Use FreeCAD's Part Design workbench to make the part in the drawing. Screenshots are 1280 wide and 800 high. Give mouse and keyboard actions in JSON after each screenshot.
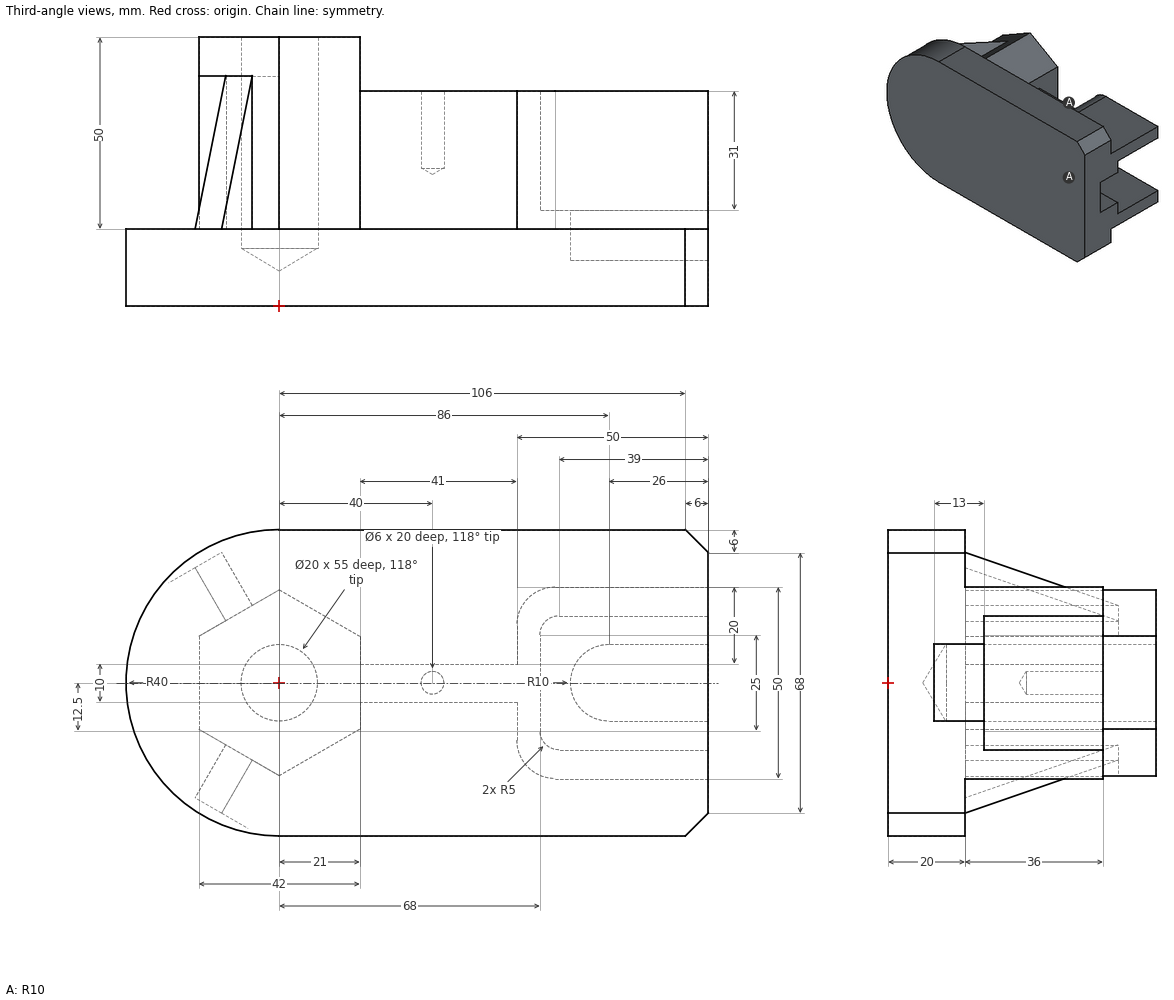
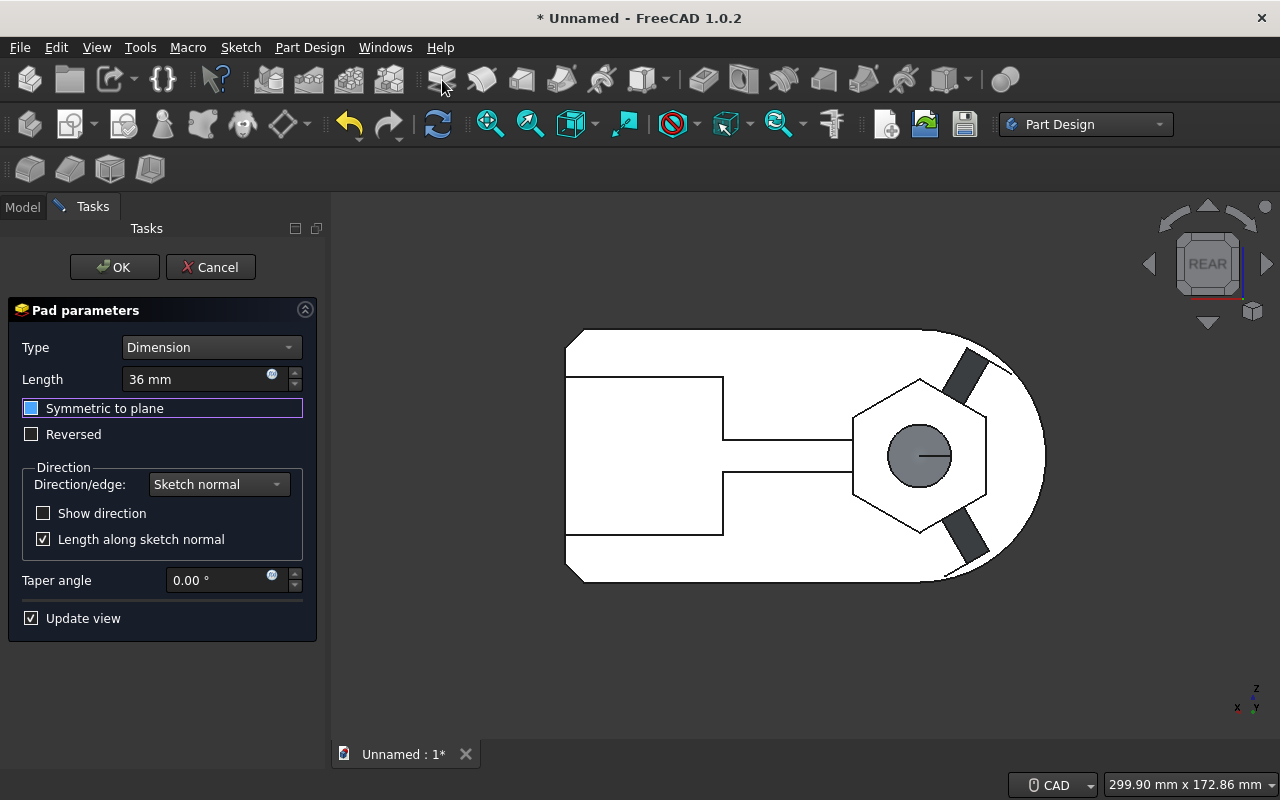
{"action": "left_click", "coordinate": [115, 267]}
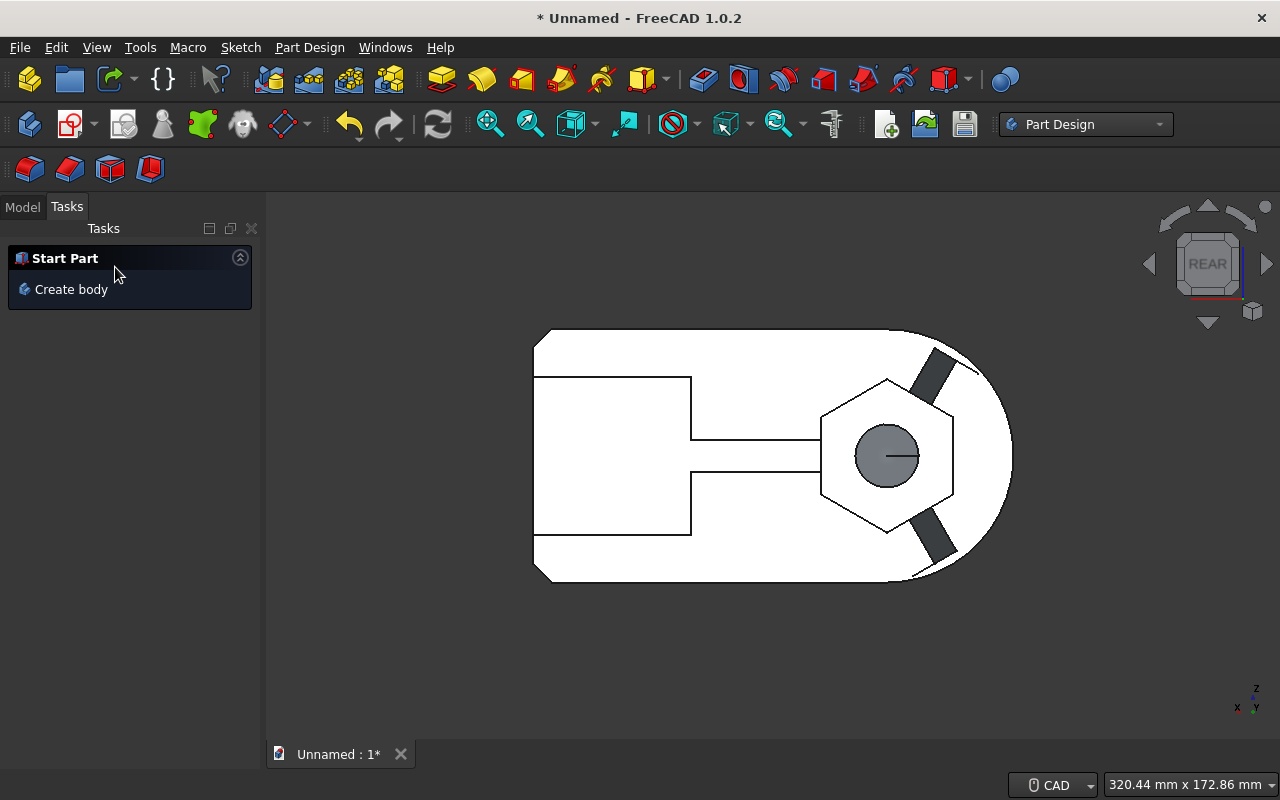
{"action": "key", "text": "0"}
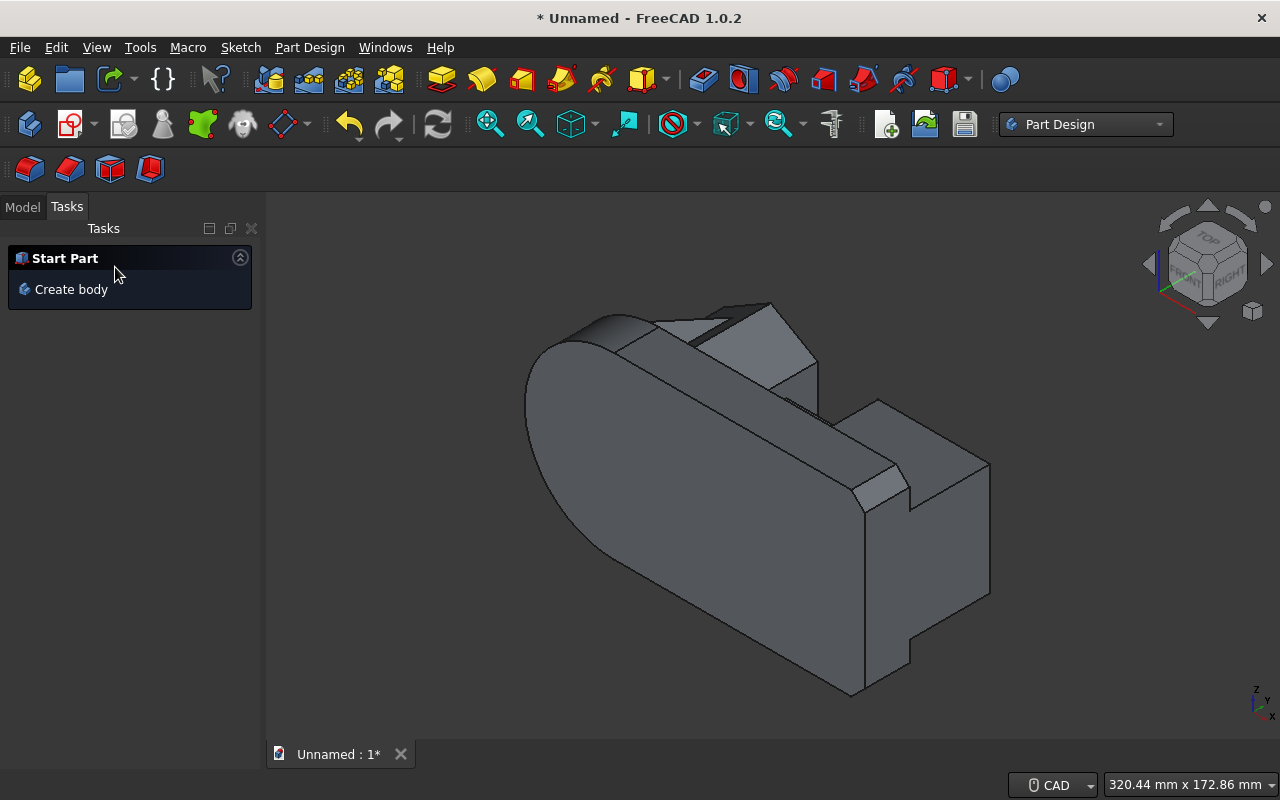
{"action": "key", "text": "2"}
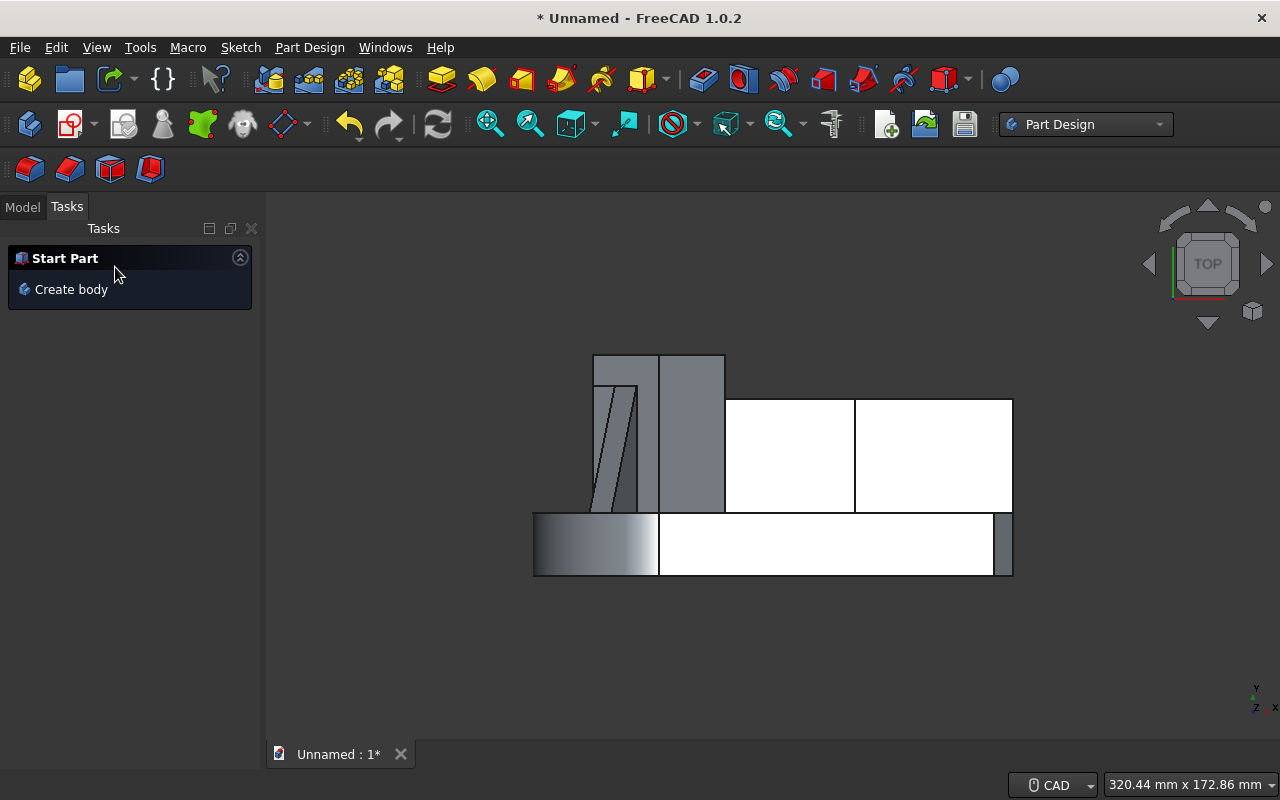
{"action": "left_click", "coordinate": [855, 455]}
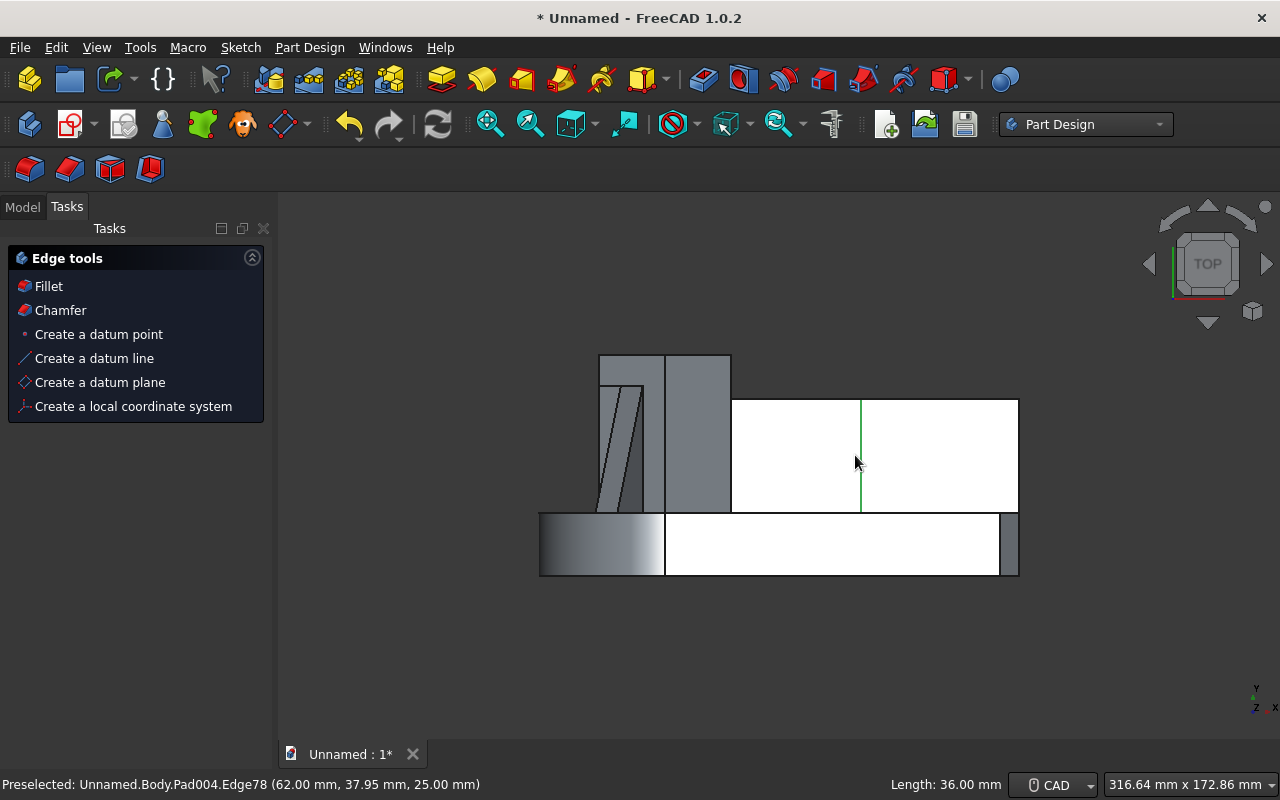
{"action": "key", "text": "1"}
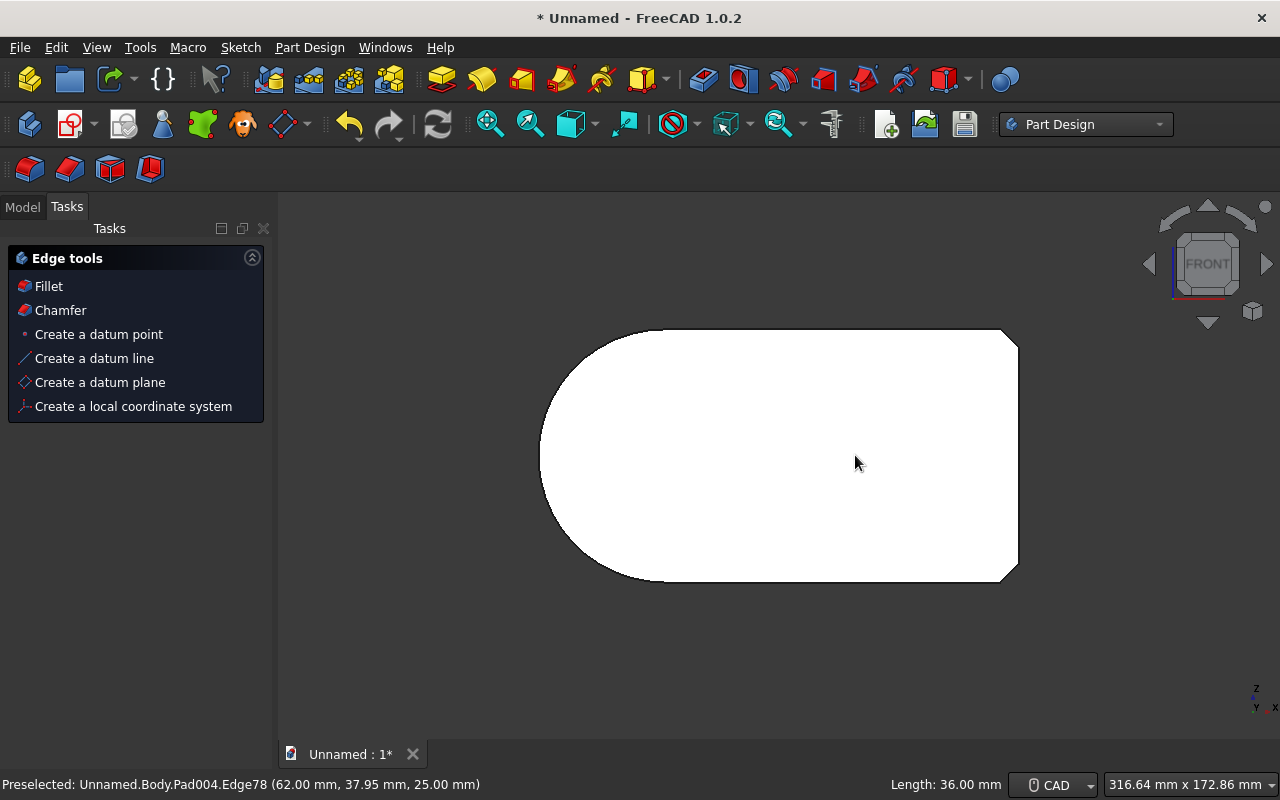
{"action": "key", "text": "3"}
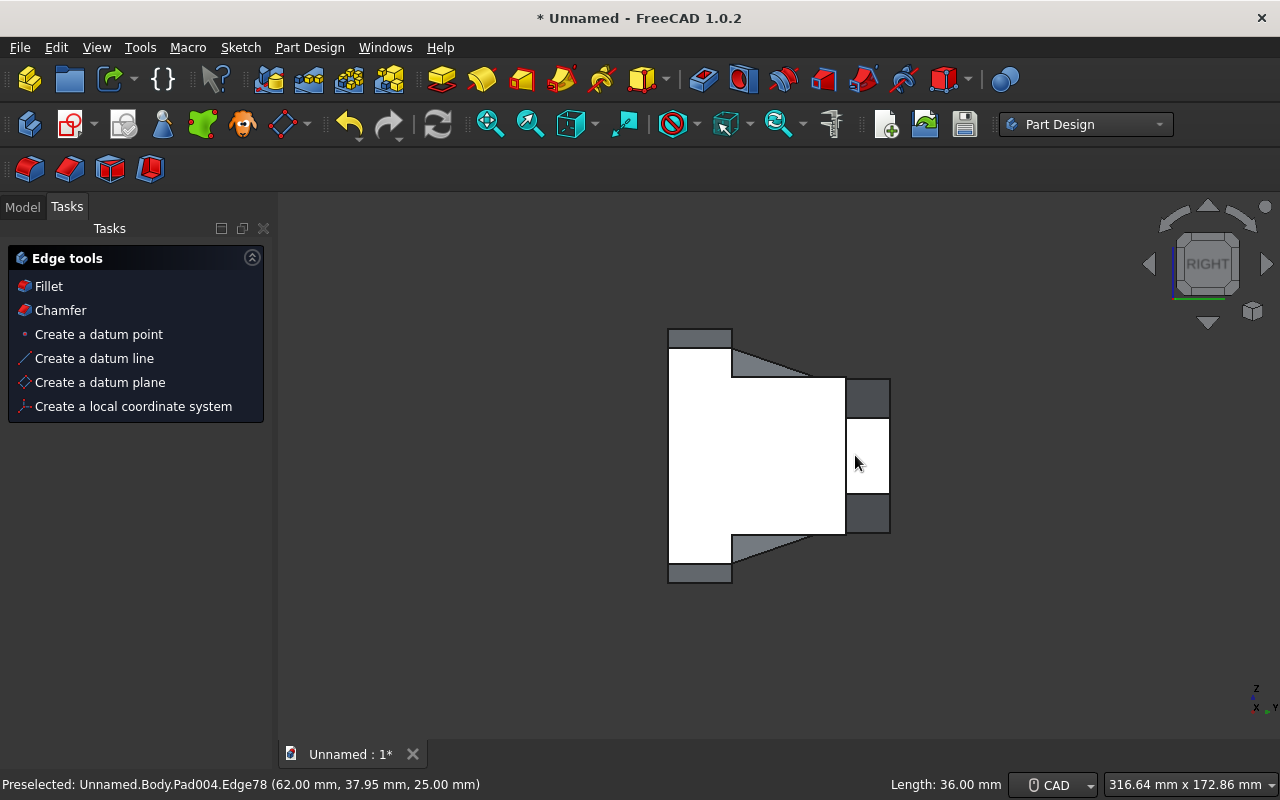
{"action": "key", "text": "5"}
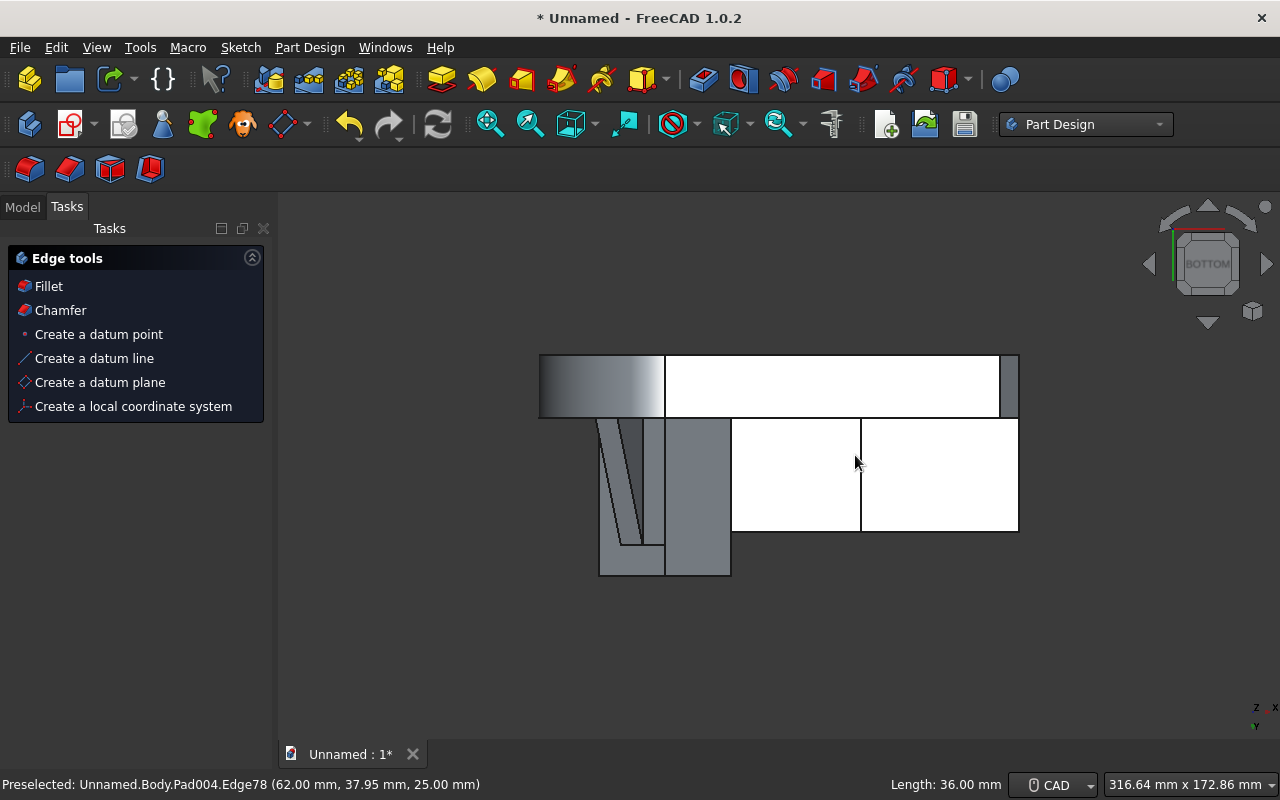
{"action": "left_click", "coordinate": [861, 474], "text": "ctrl"}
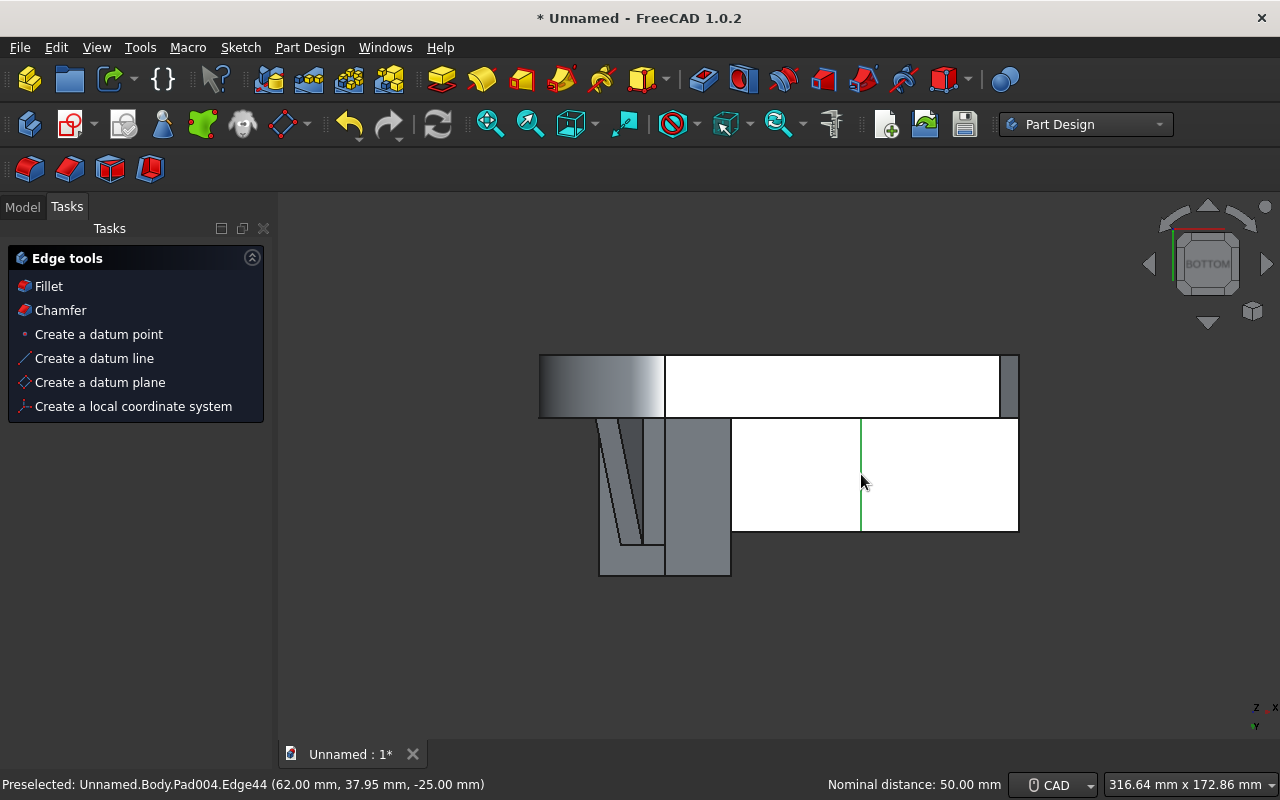
{"action": "left_click", "coordinate": [30, 170]}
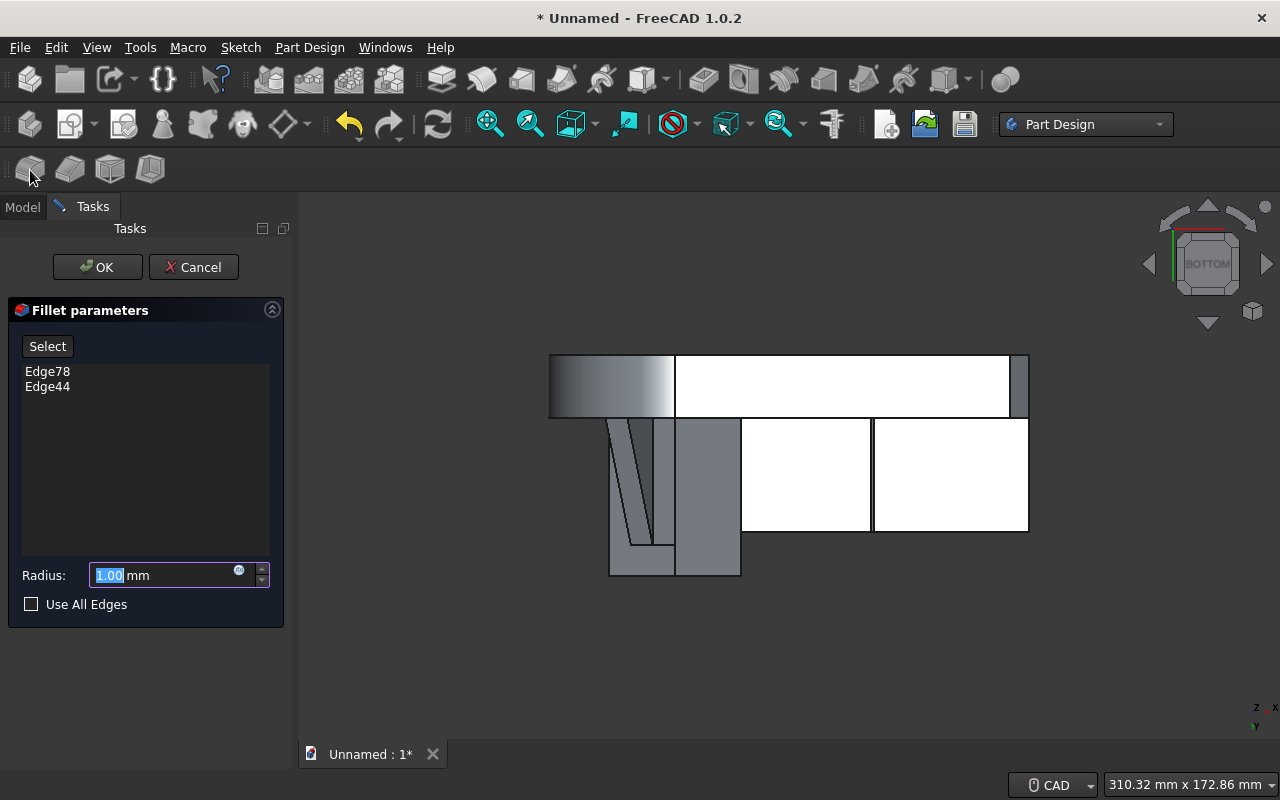
{"action": "type", "text": "10"}
{"action": "key", "text": "Tab"}